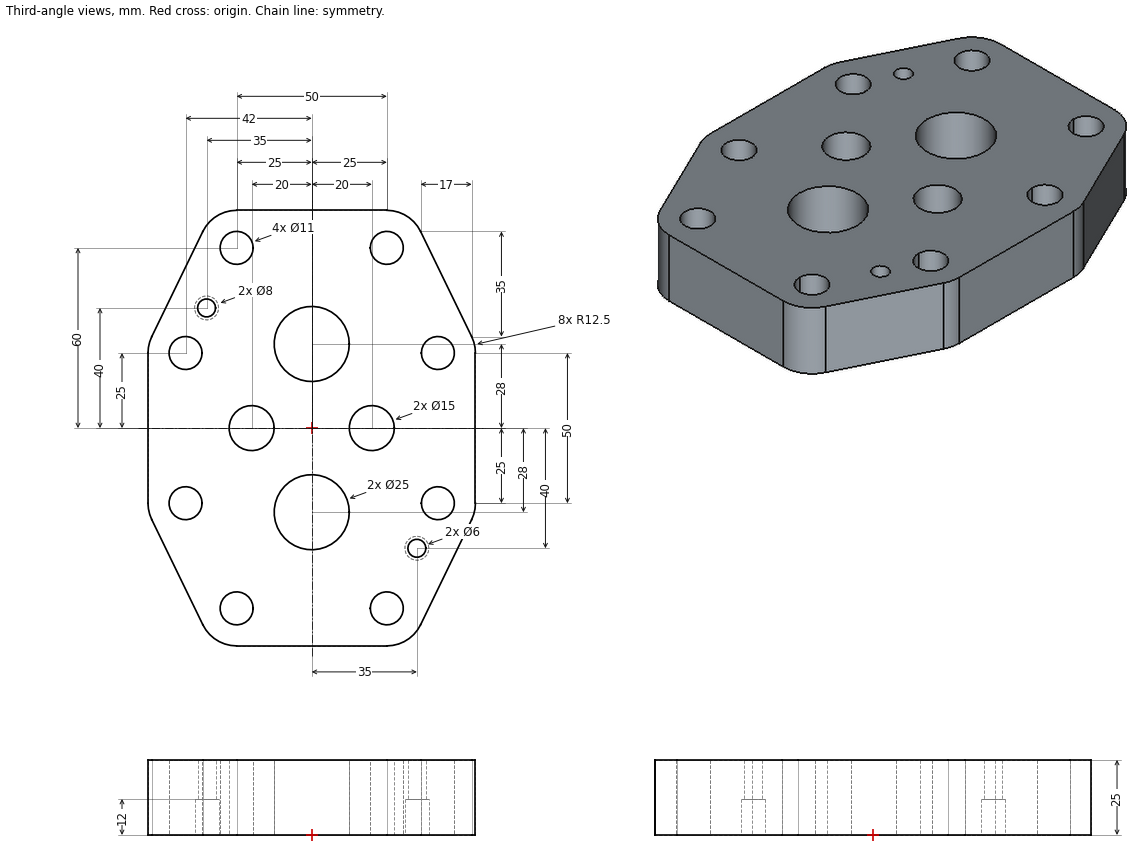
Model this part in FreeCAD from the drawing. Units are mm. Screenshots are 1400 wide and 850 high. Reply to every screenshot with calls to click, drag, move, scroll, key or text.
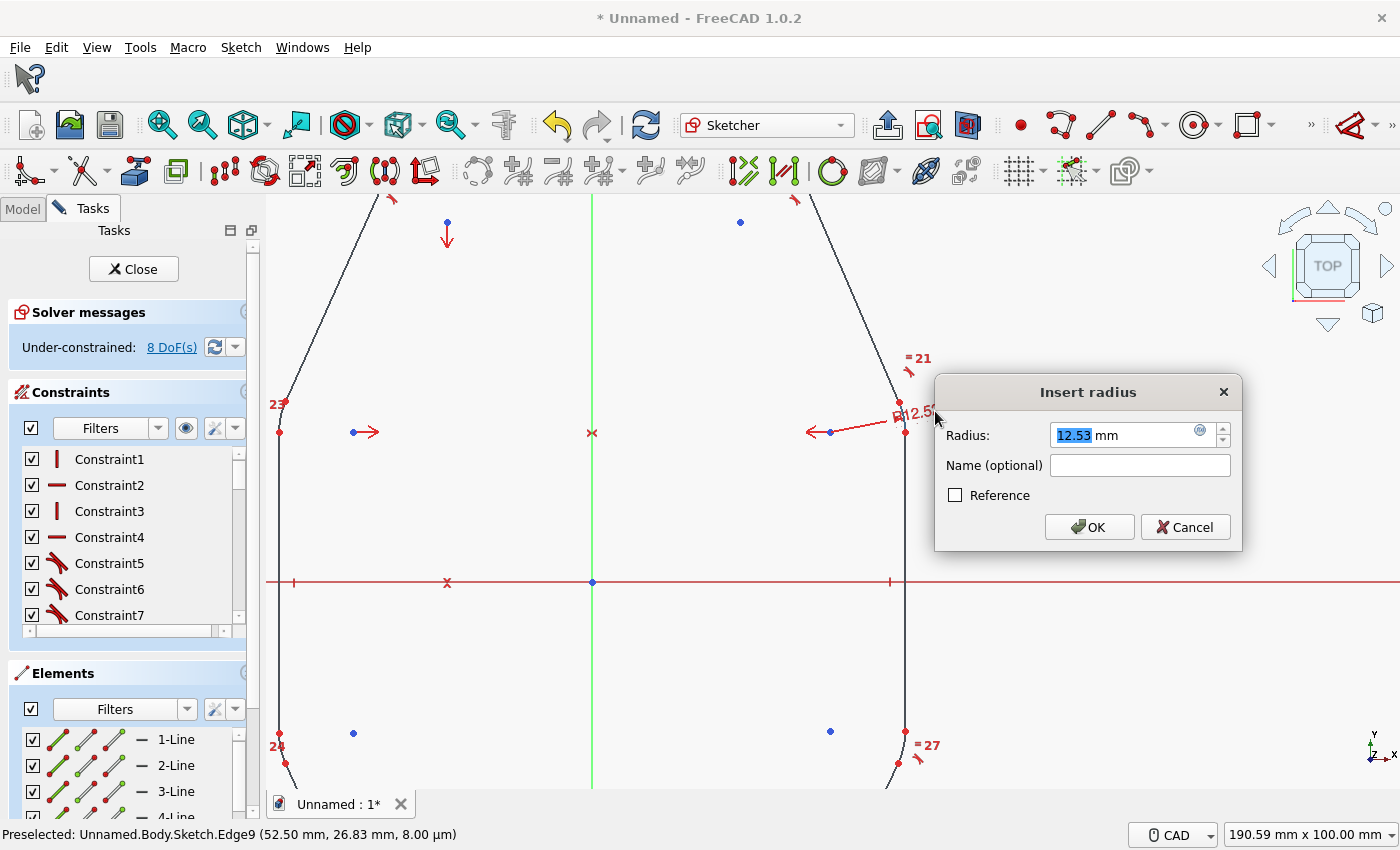
text(12.5)
key(Return)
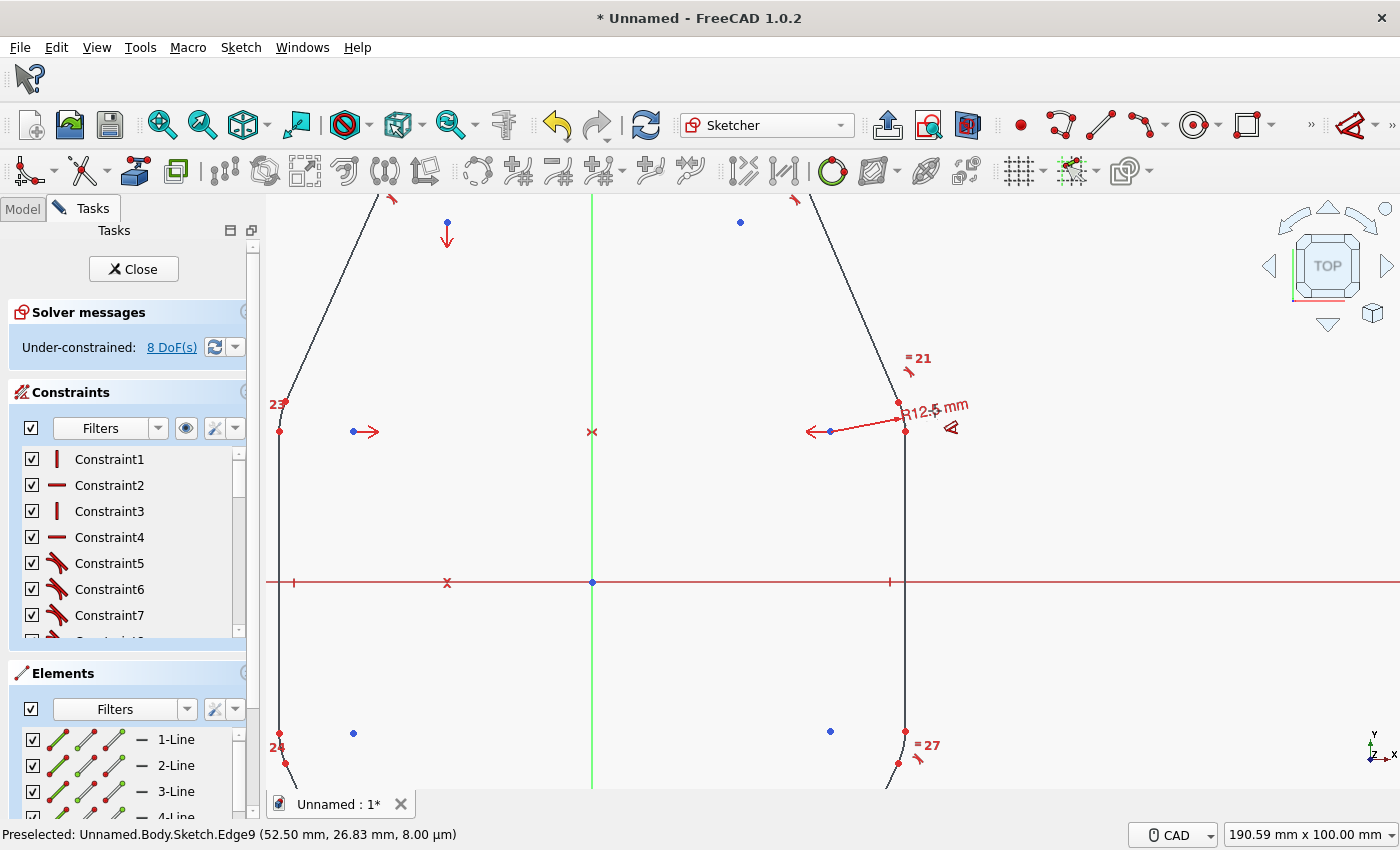
click(905, 642)
click(939, 513)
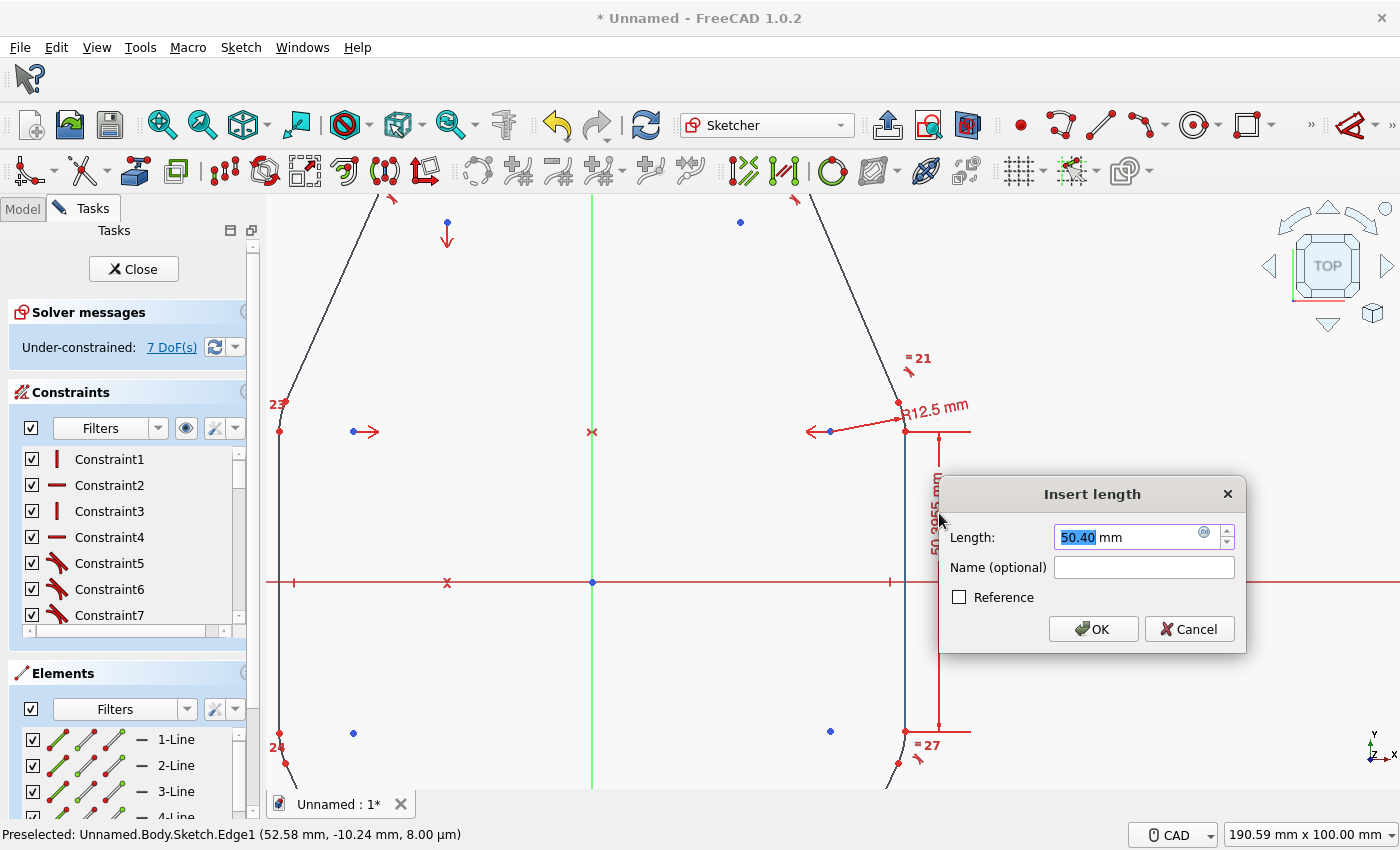
text(50)
key(Return)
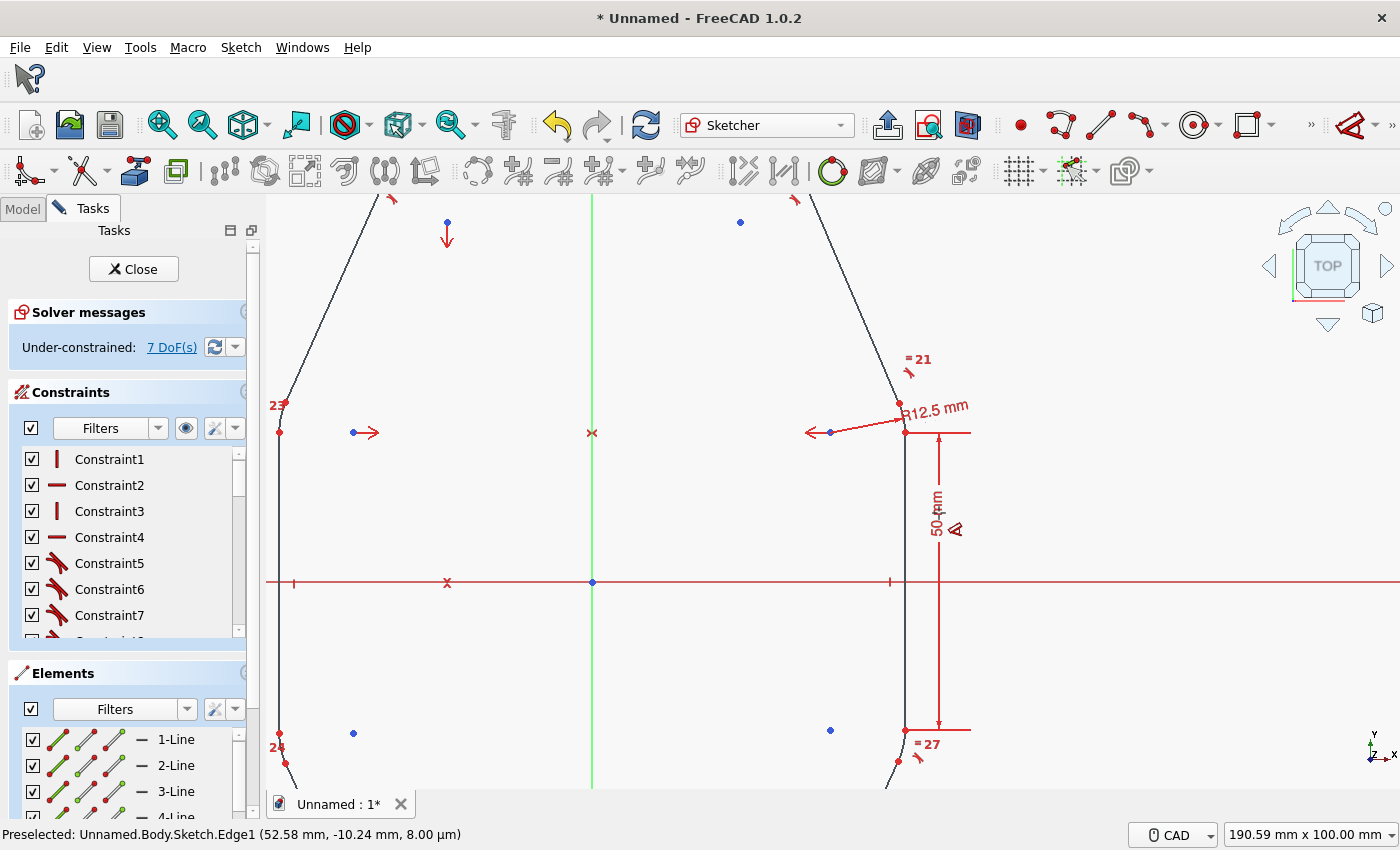
scroll(905, 418, down, 4)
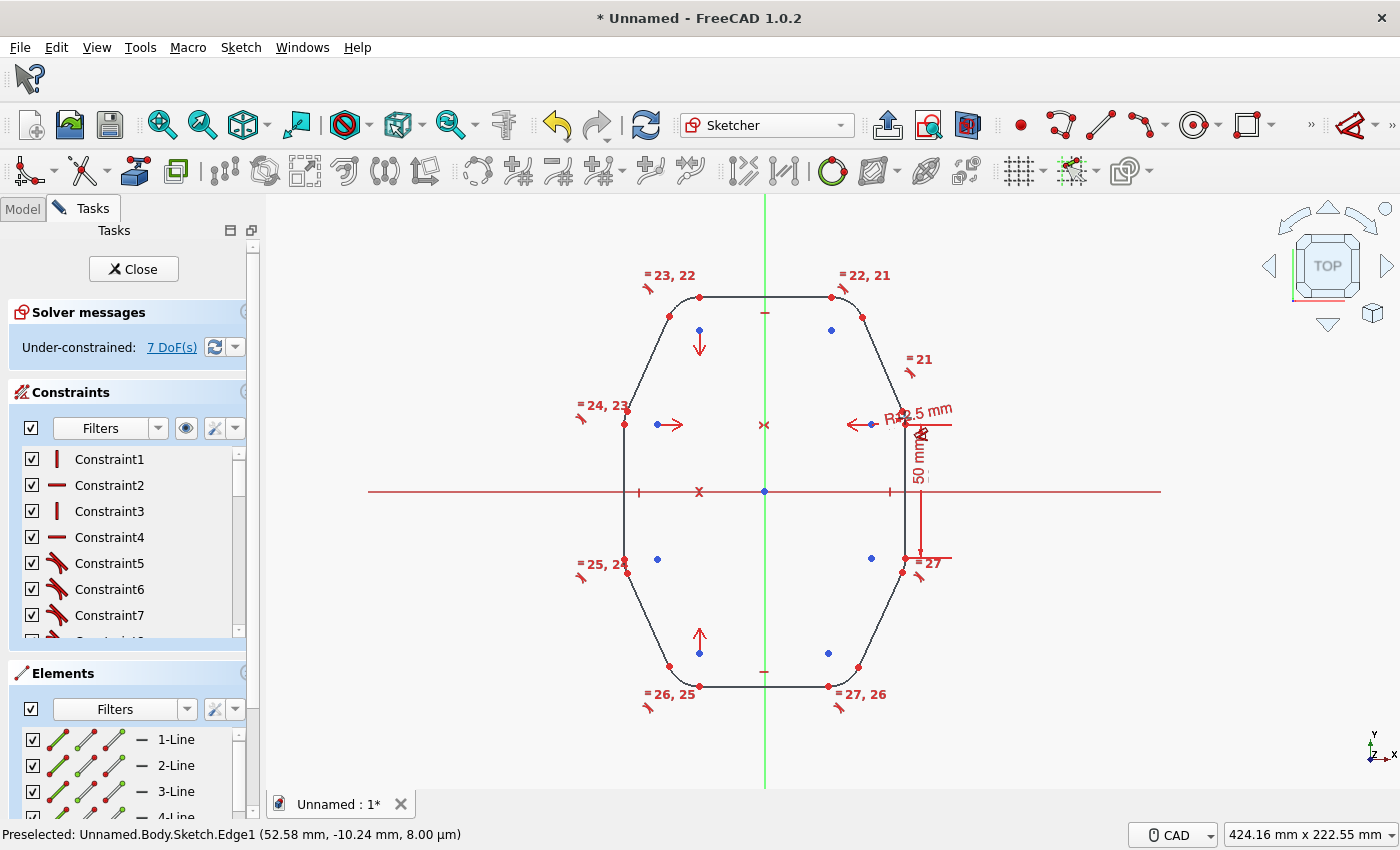
click(792, 297)
click(735, 263)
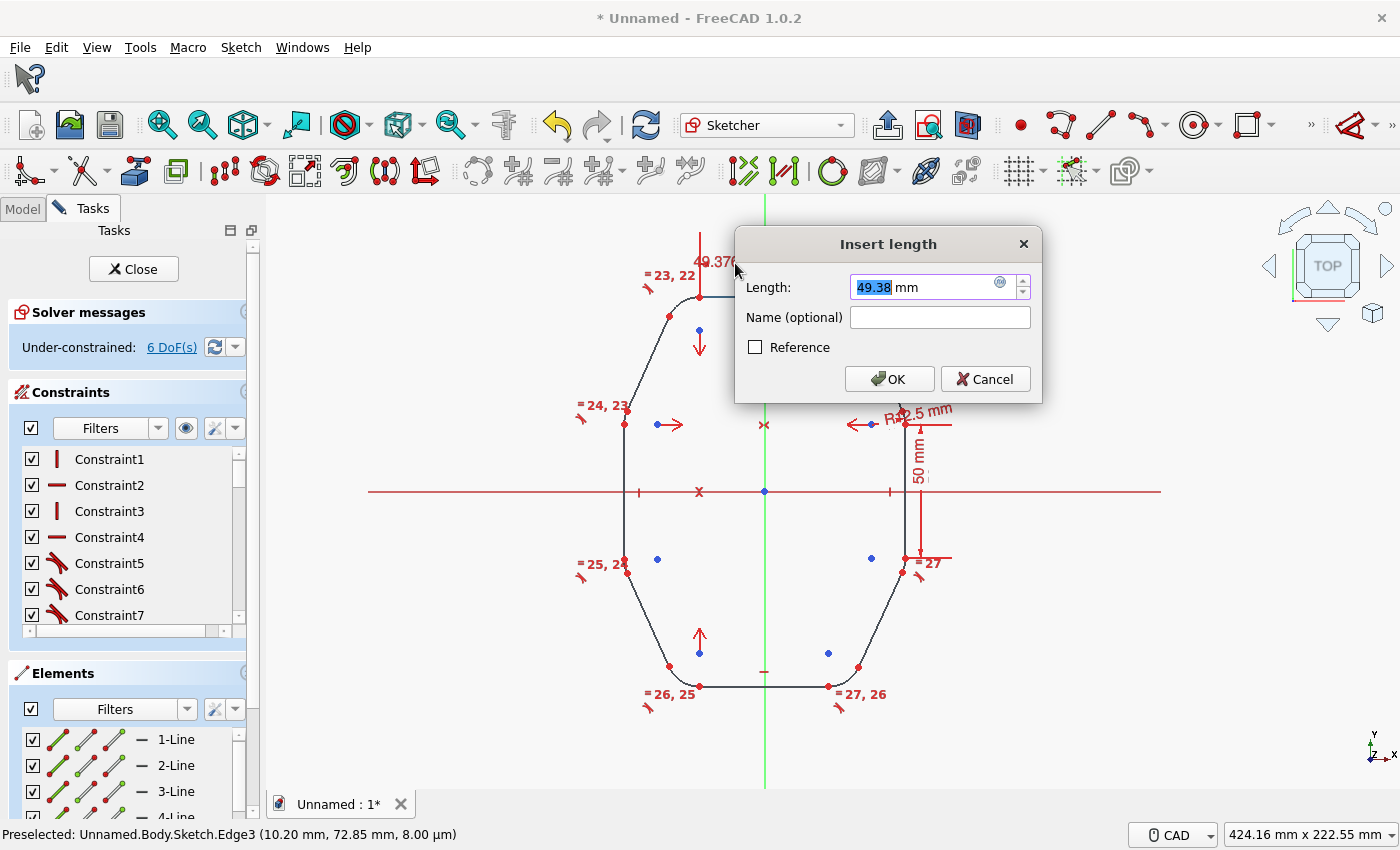
text(50)
key(Return)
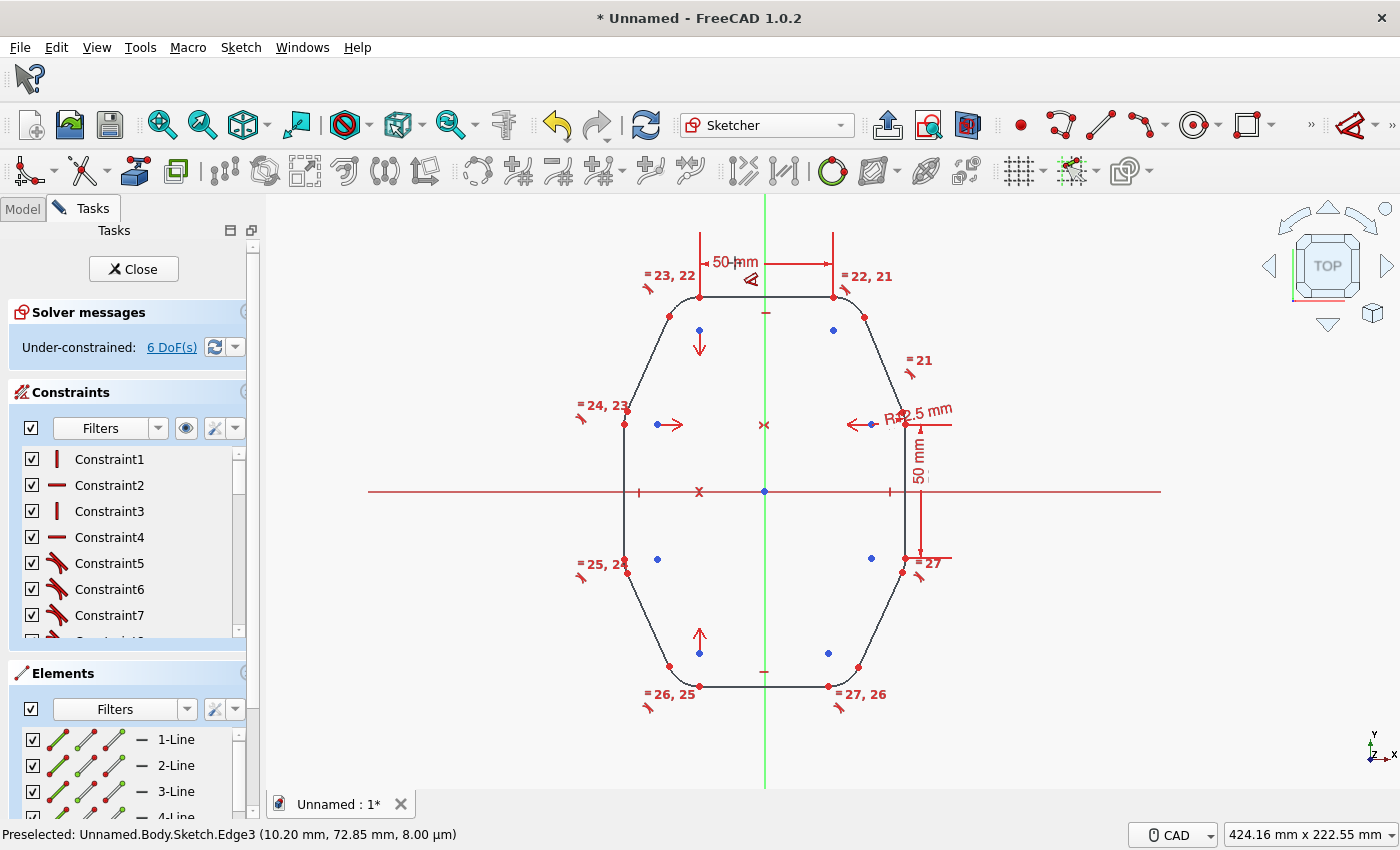
click(624, 465)
click(590, 461)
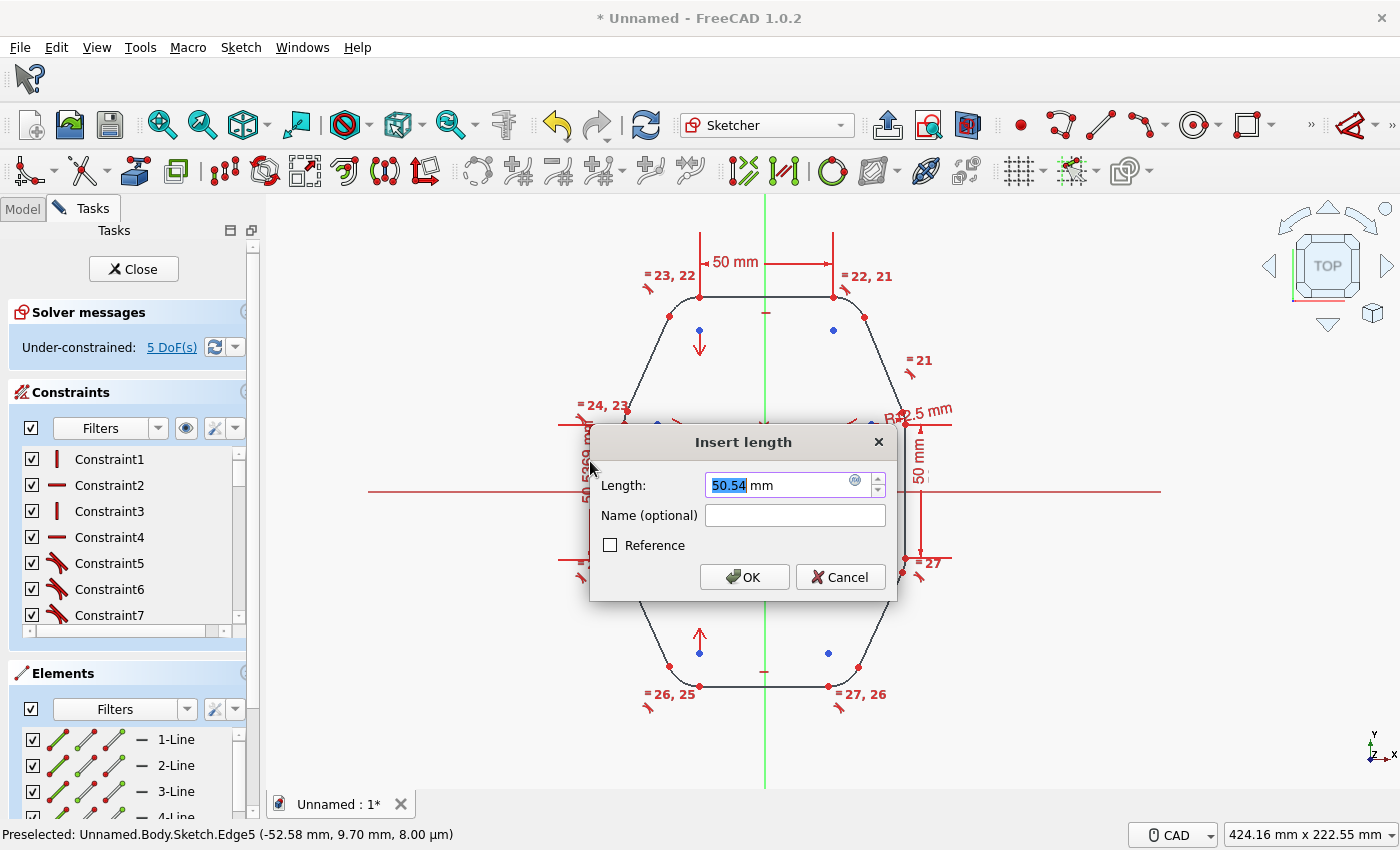
text(50)
key(Return)